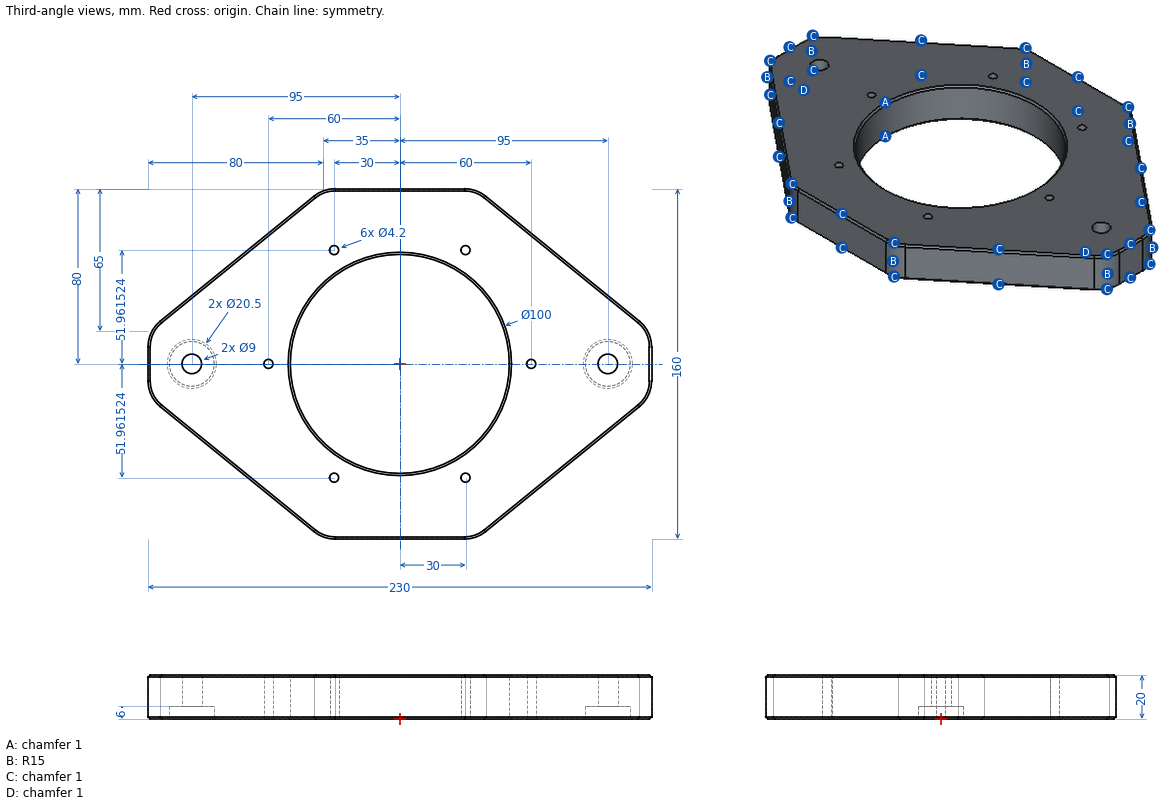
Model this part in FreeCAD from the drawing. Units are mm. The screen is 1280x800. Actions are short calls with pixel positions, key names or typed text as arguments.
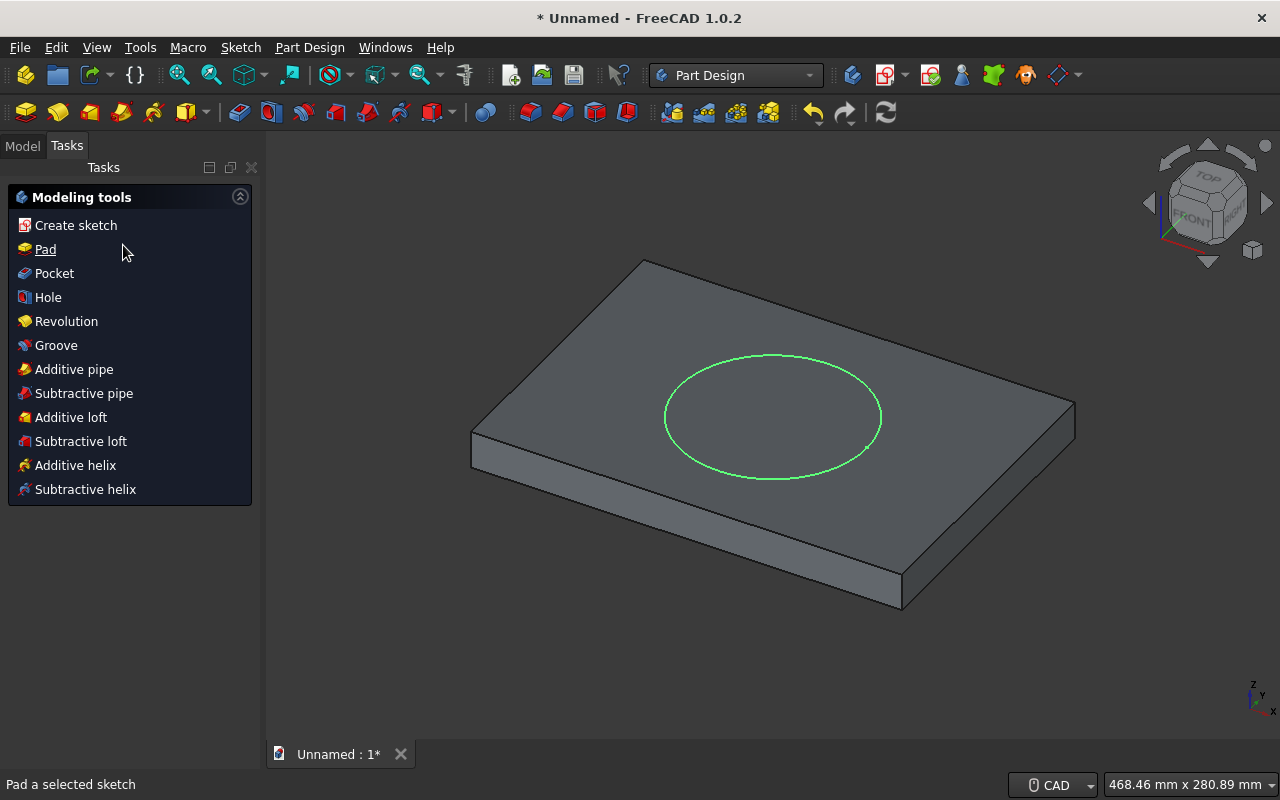
click(240, 112)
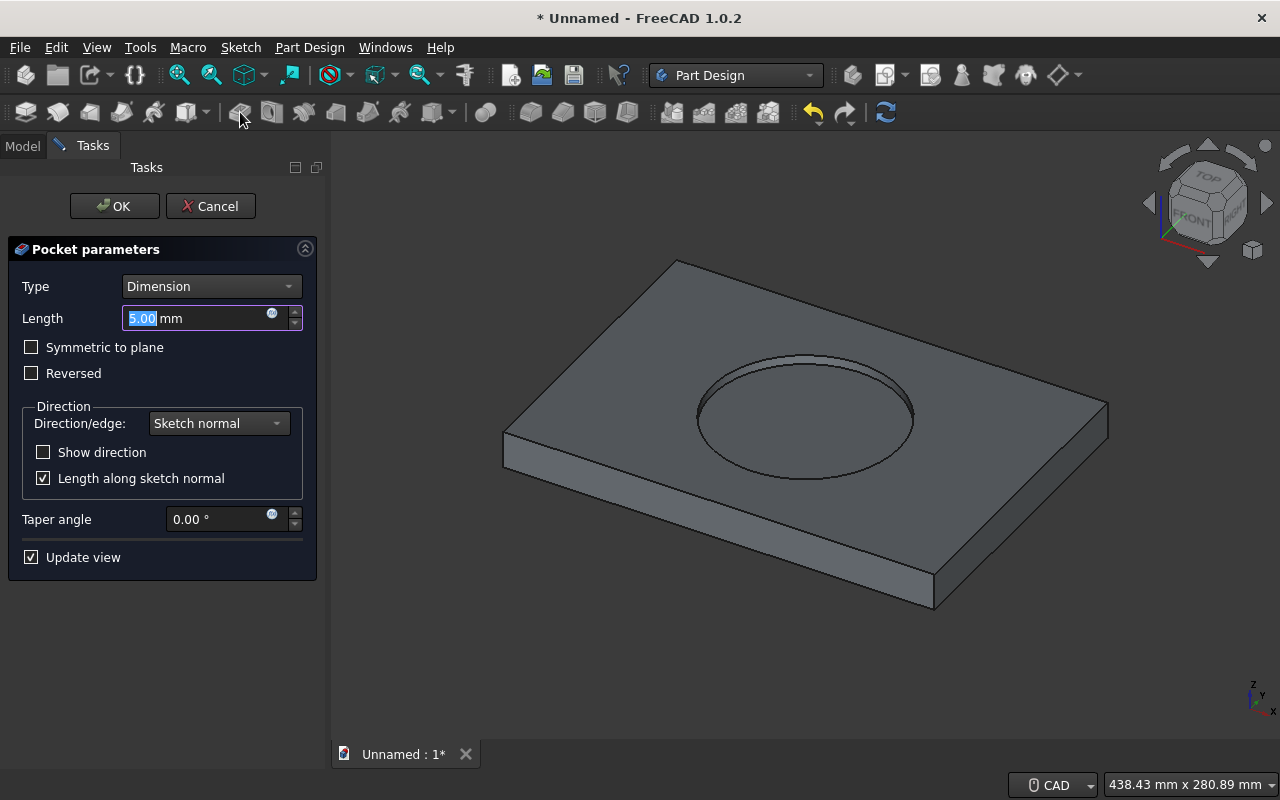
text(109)
key(Tab)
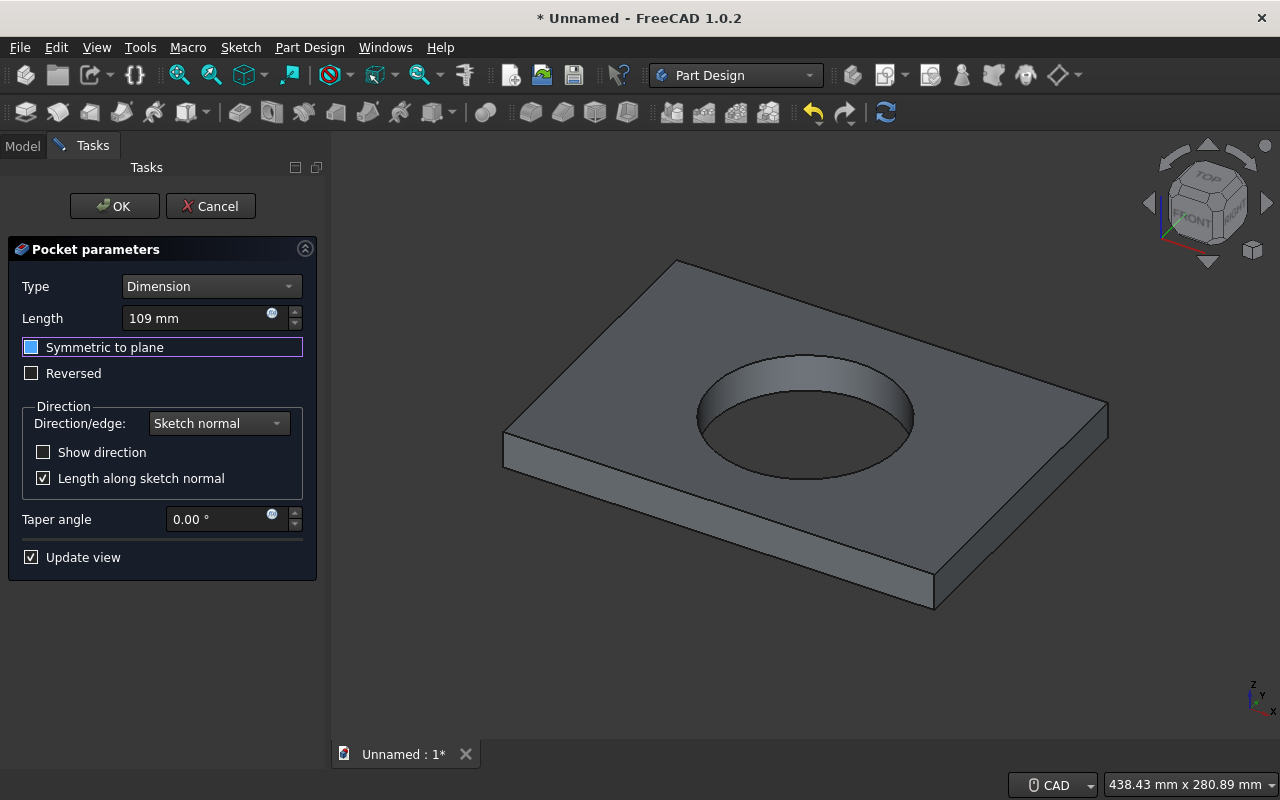
click(115, 206)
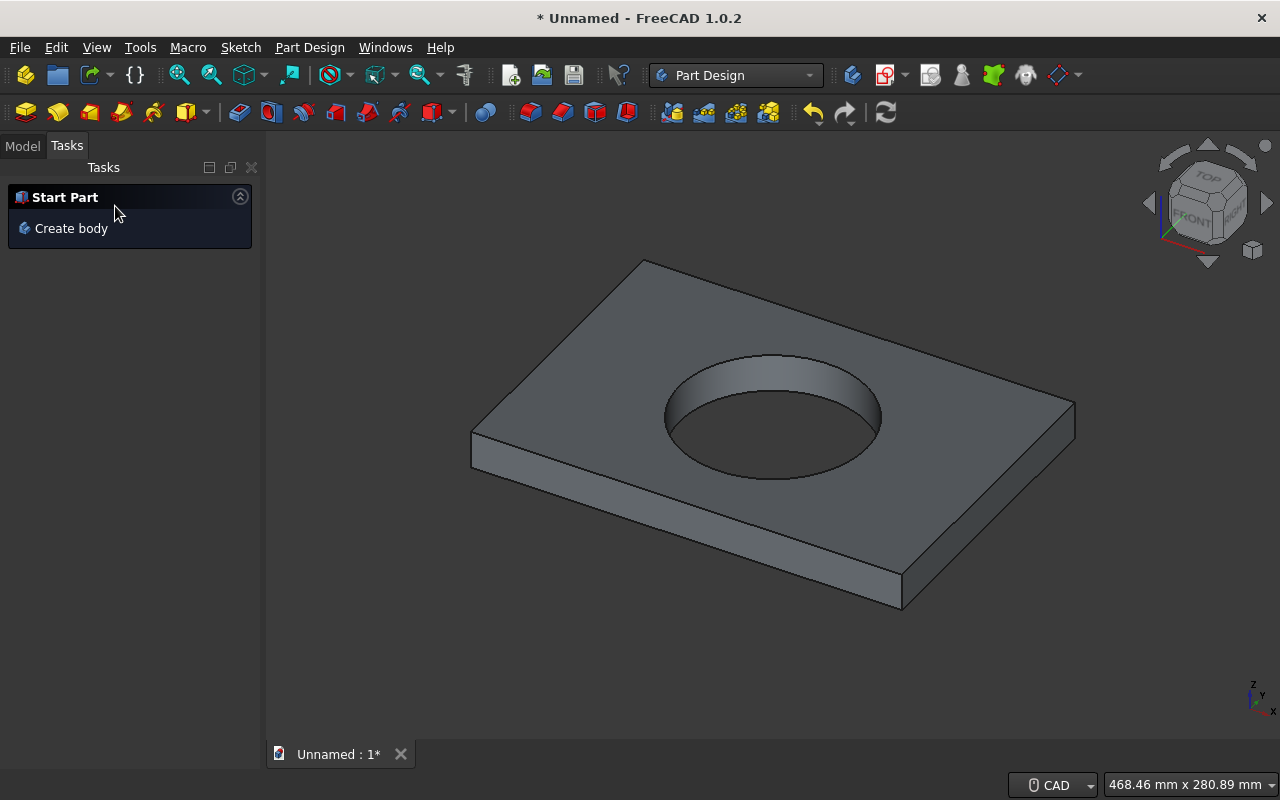
click(886, 76)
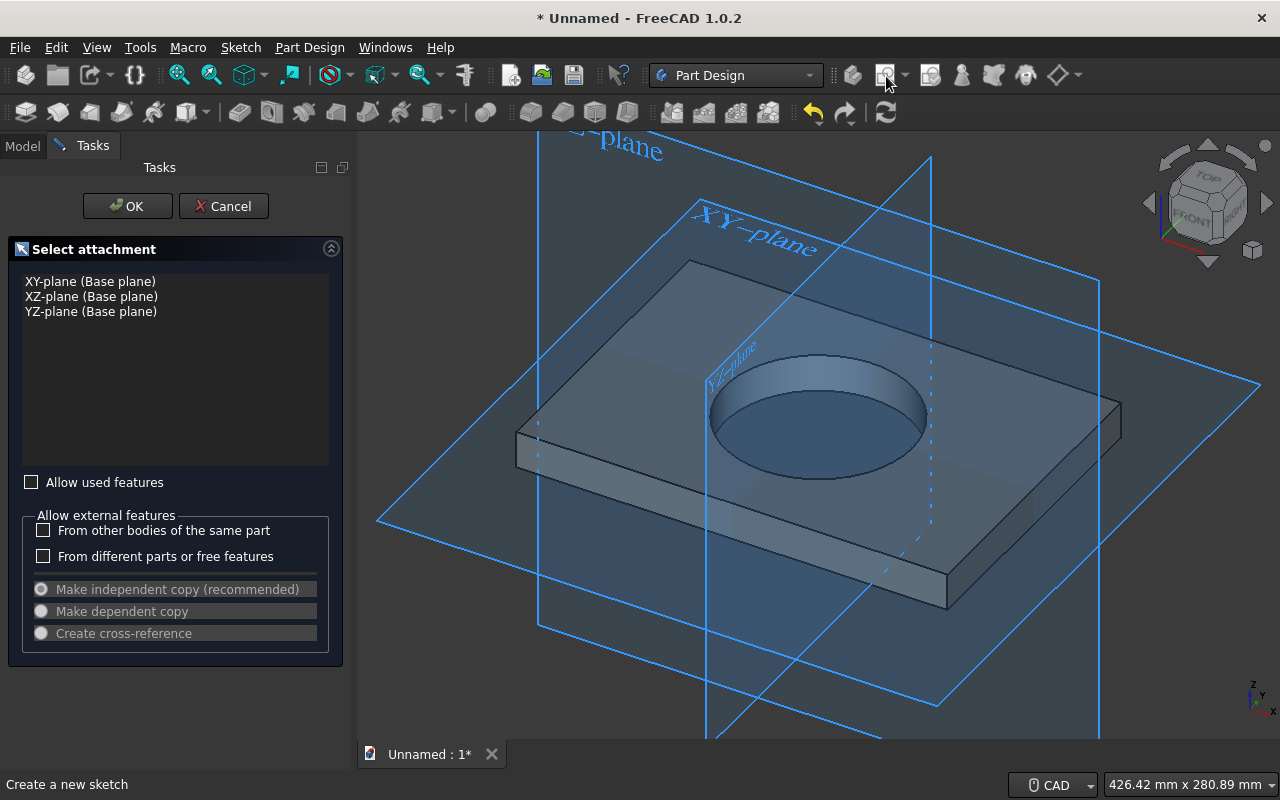
click(82, 282)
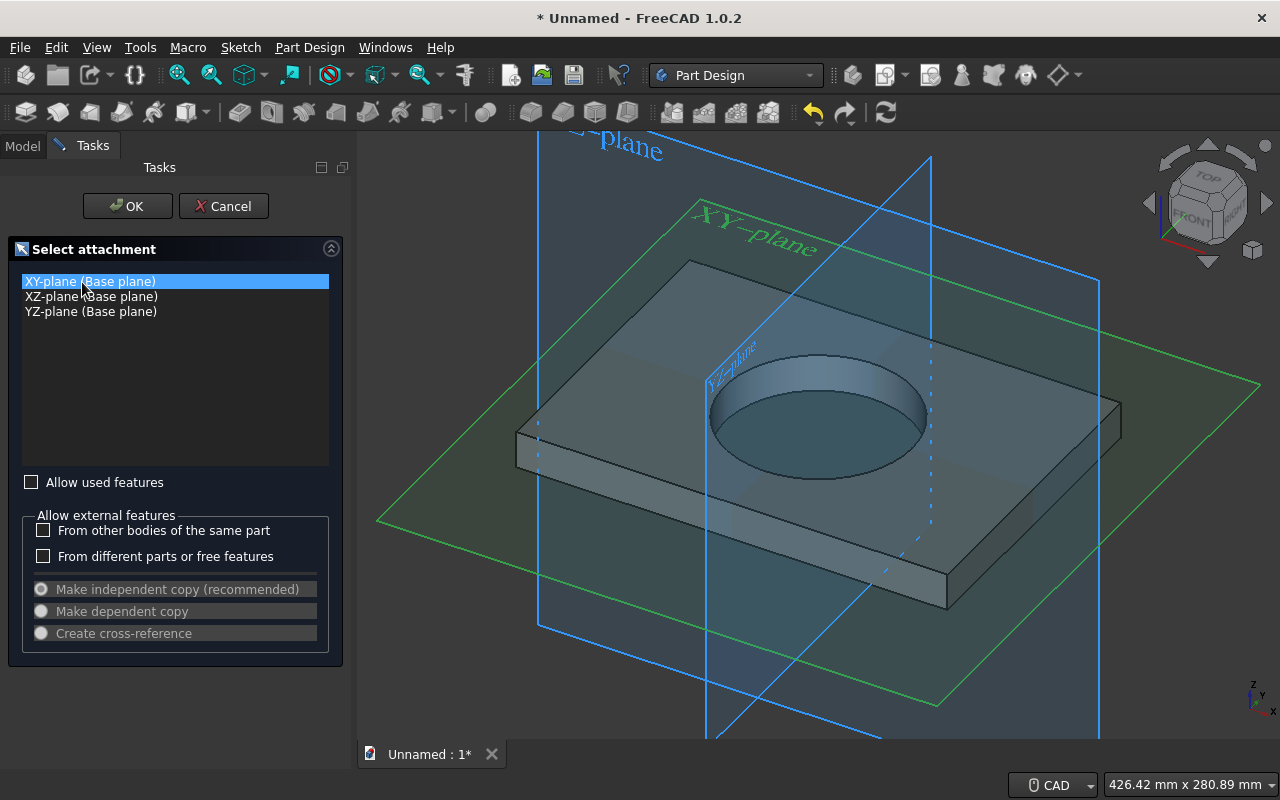
click(128, 206)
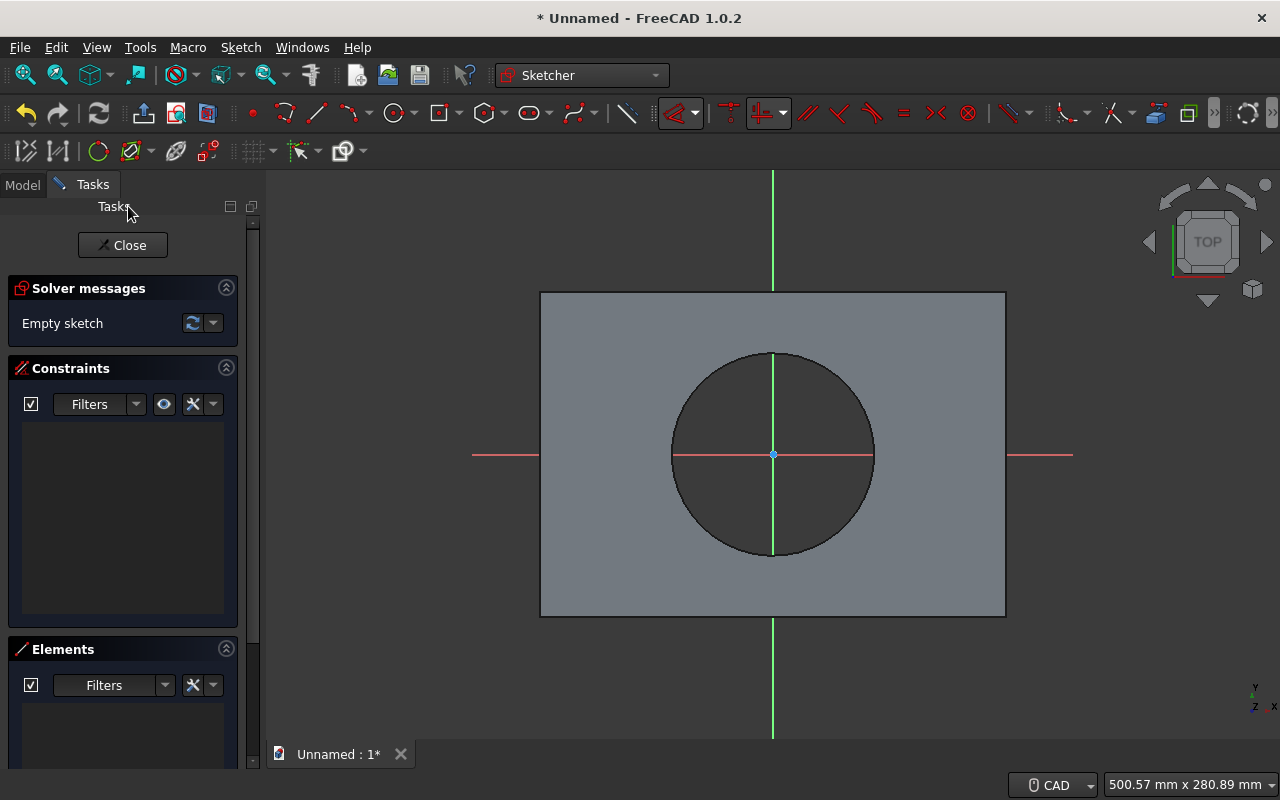
click(208, 114)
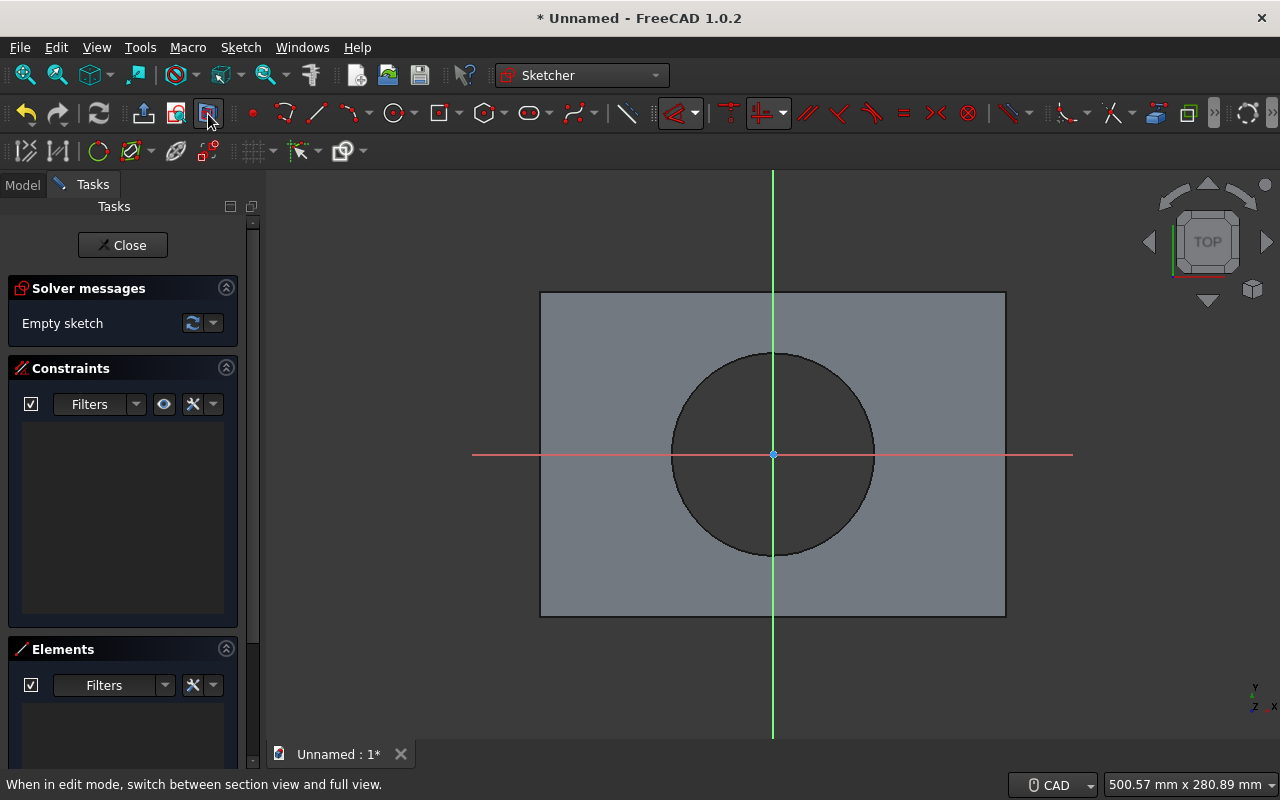
scroll(912, 455, up, 2)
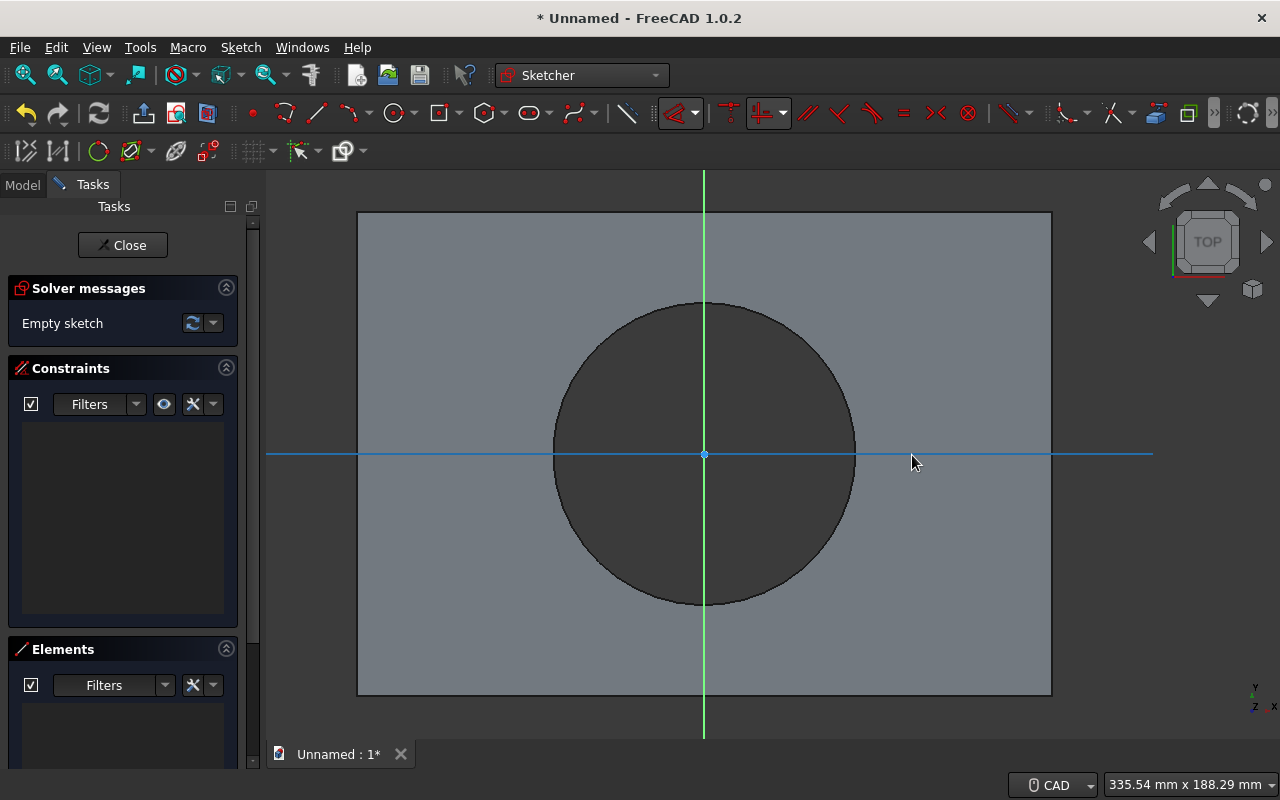
click(394, 114)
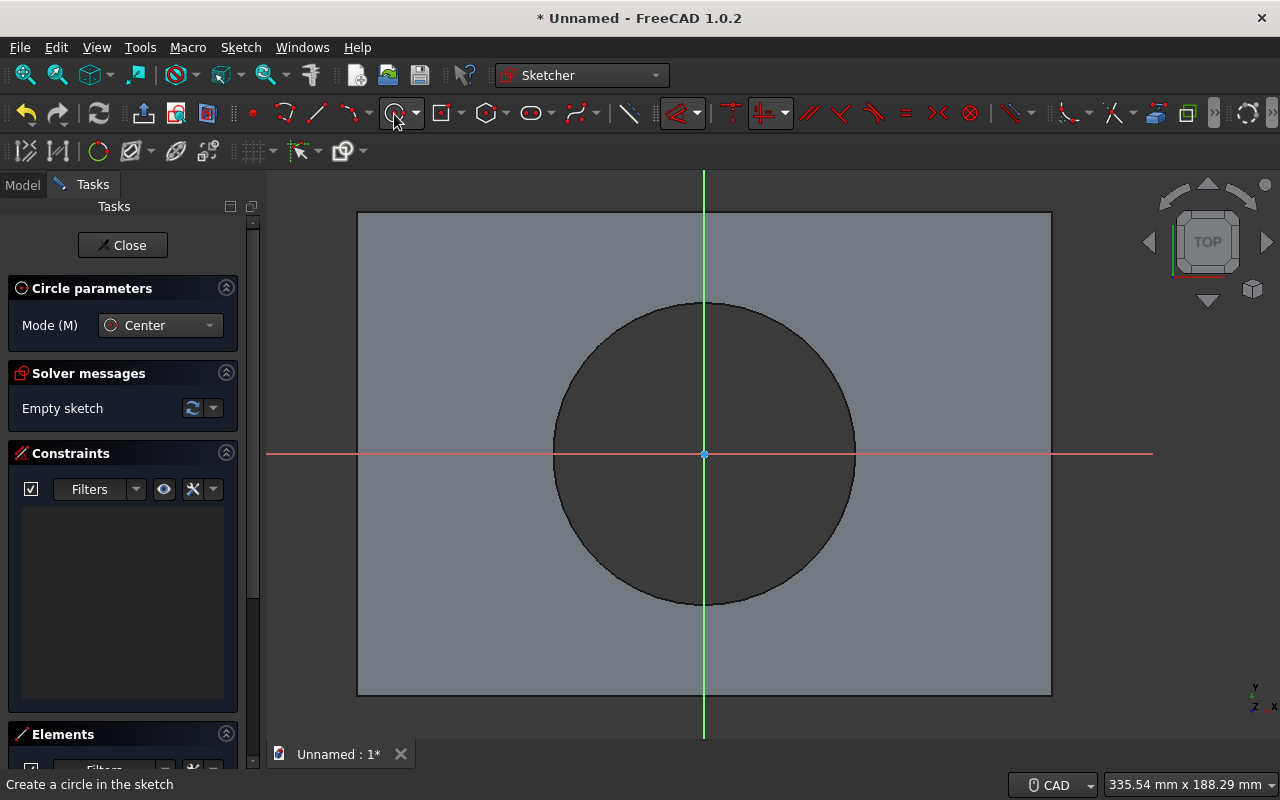
click(417, 454)
move(439, 432)